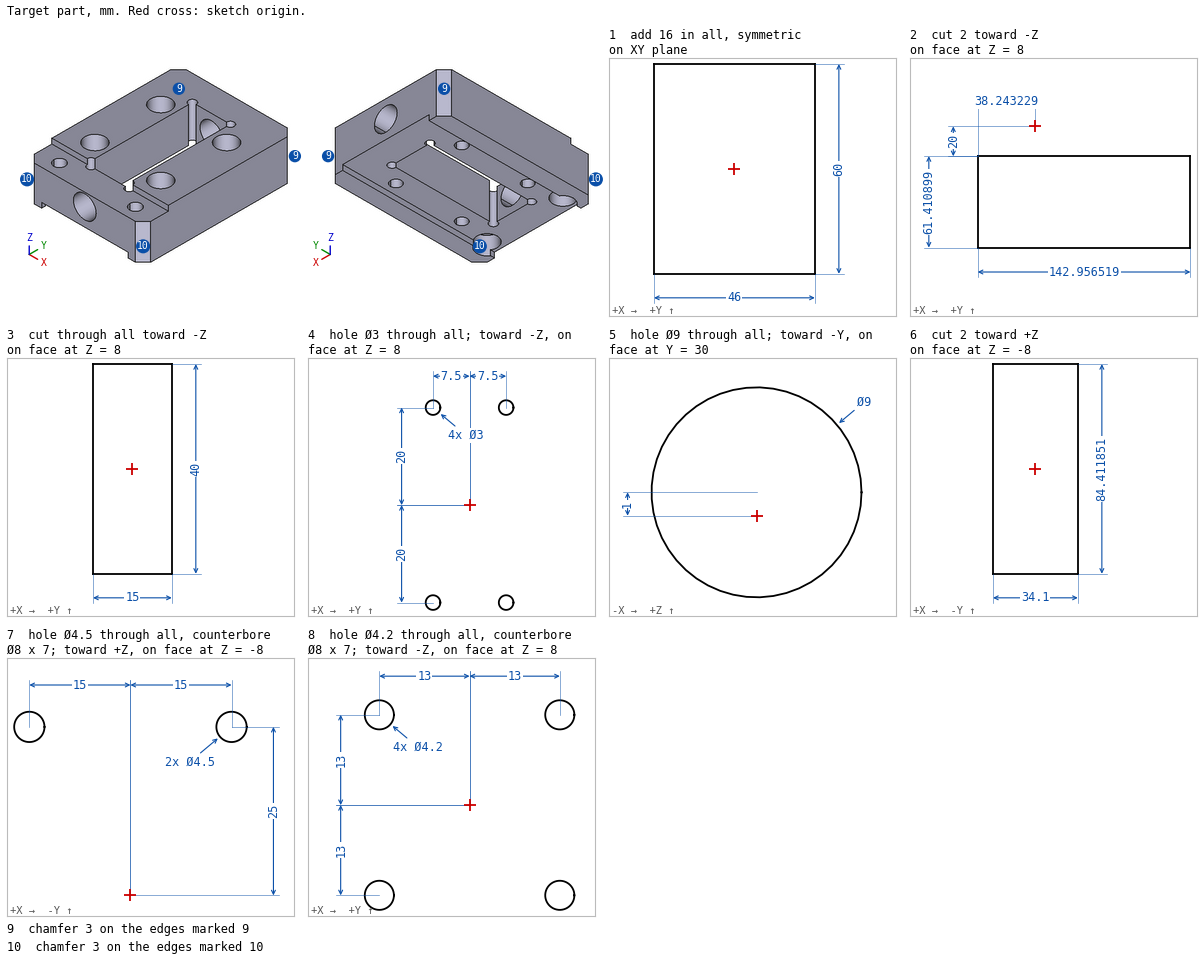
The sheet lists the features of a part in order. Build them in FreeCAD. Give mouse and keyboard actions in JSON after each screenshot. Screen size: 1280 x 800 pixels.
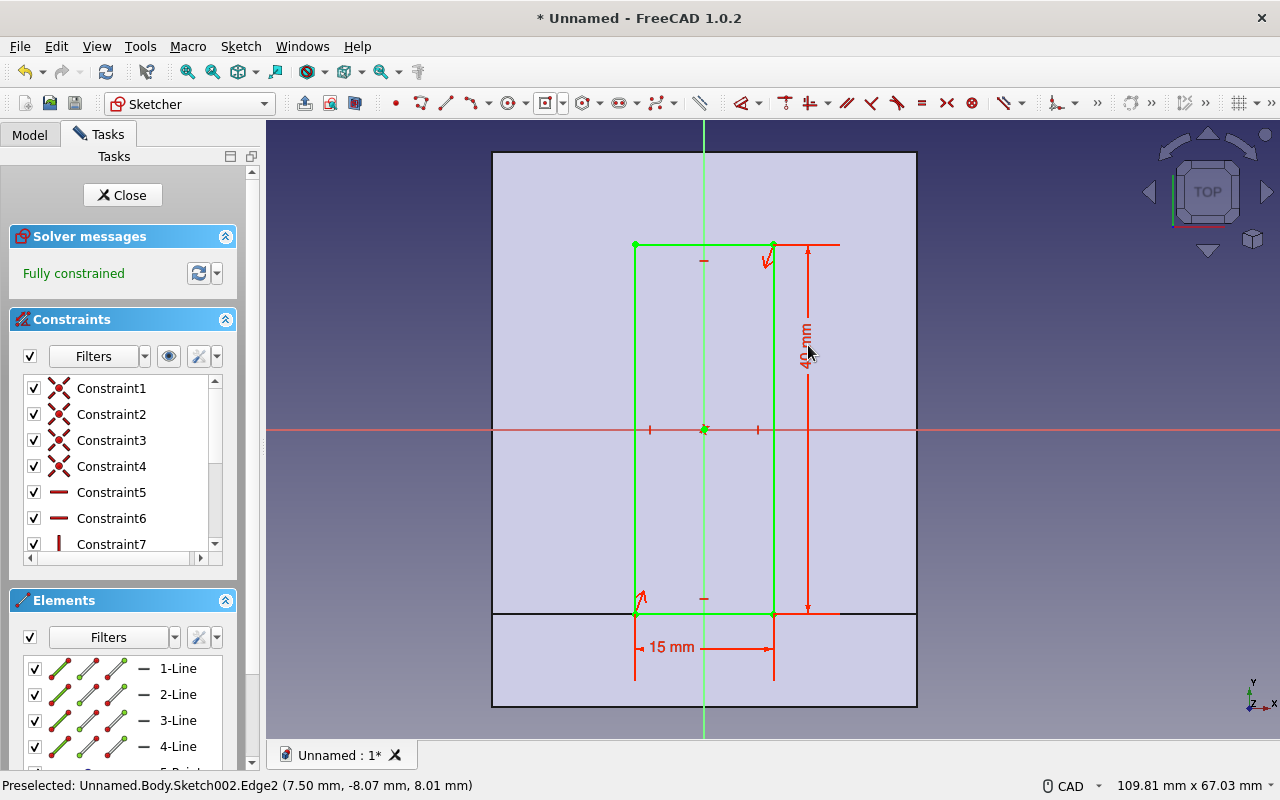
{"action": "left_click", "coordinate": [123, 195]}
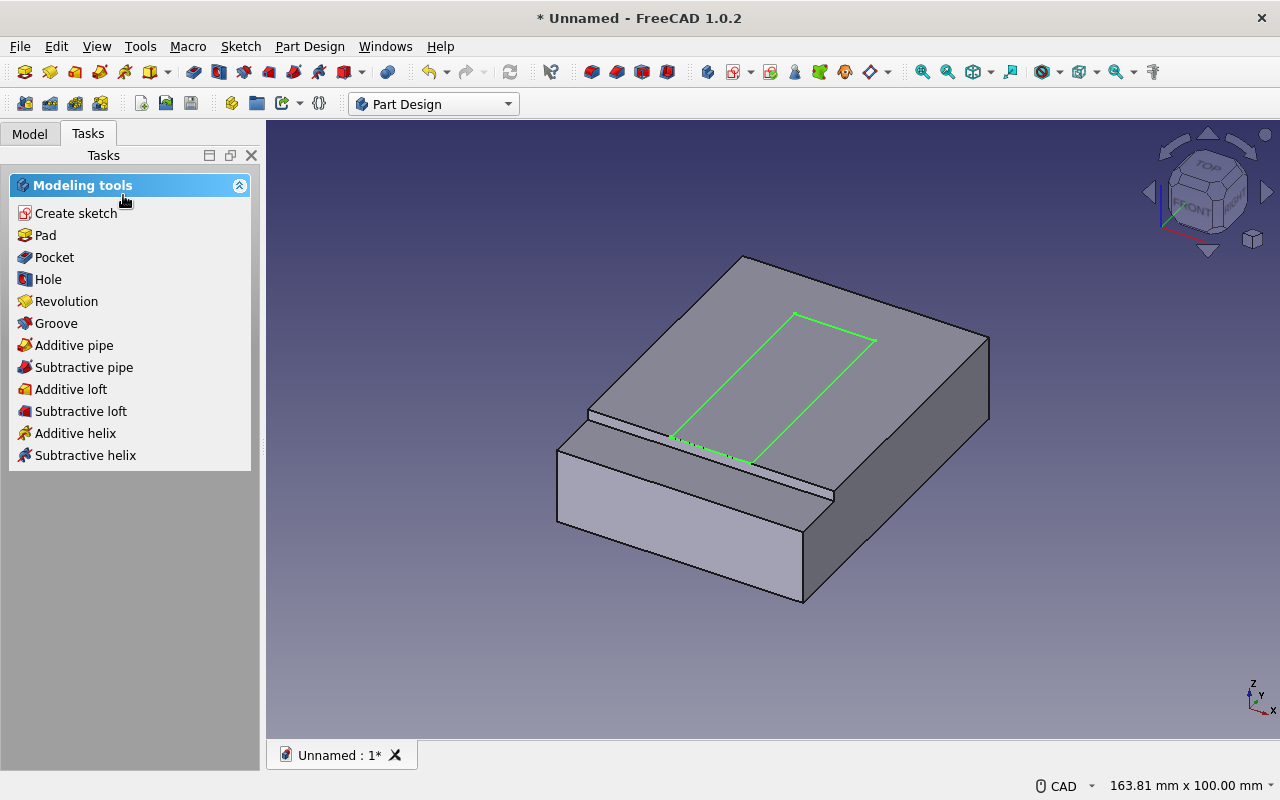
{"action": "left_click", "coordinate": [194, 72]}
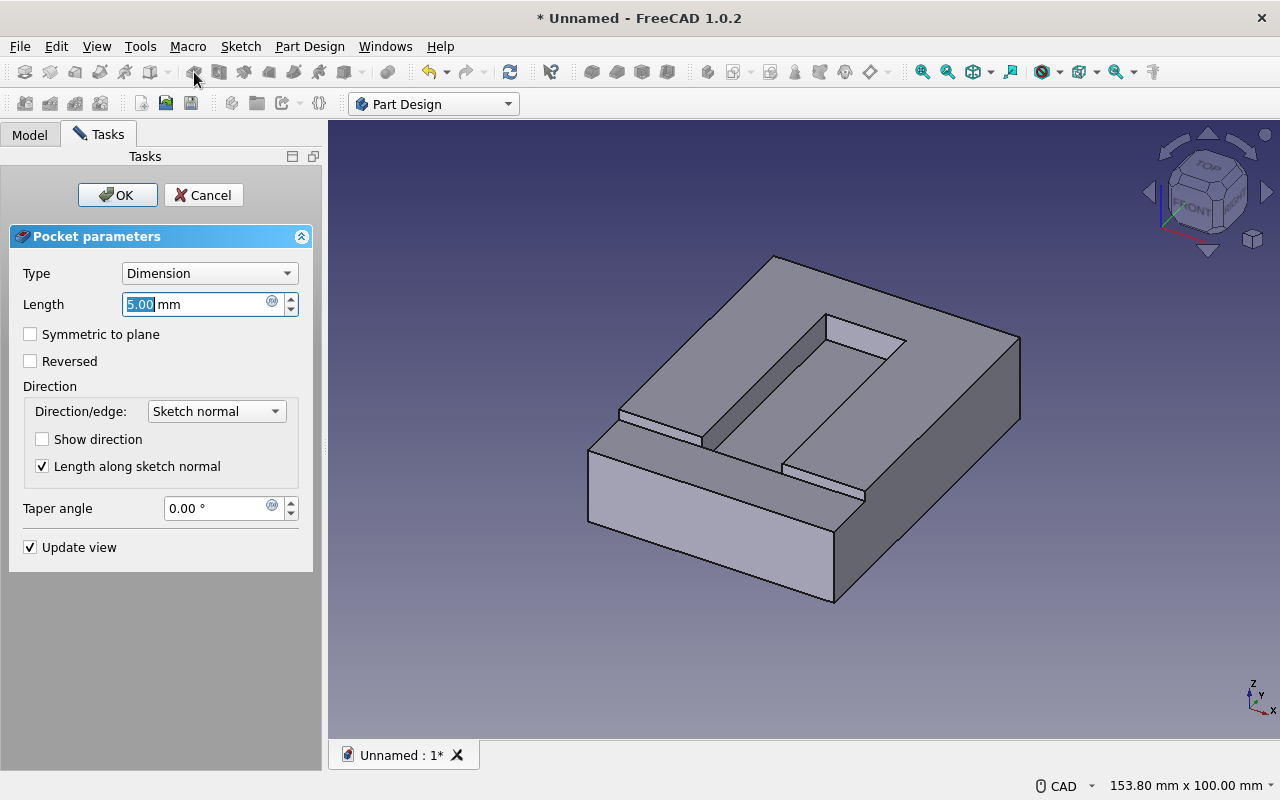
{"action": "left_click", "coordinate": [210, 274]}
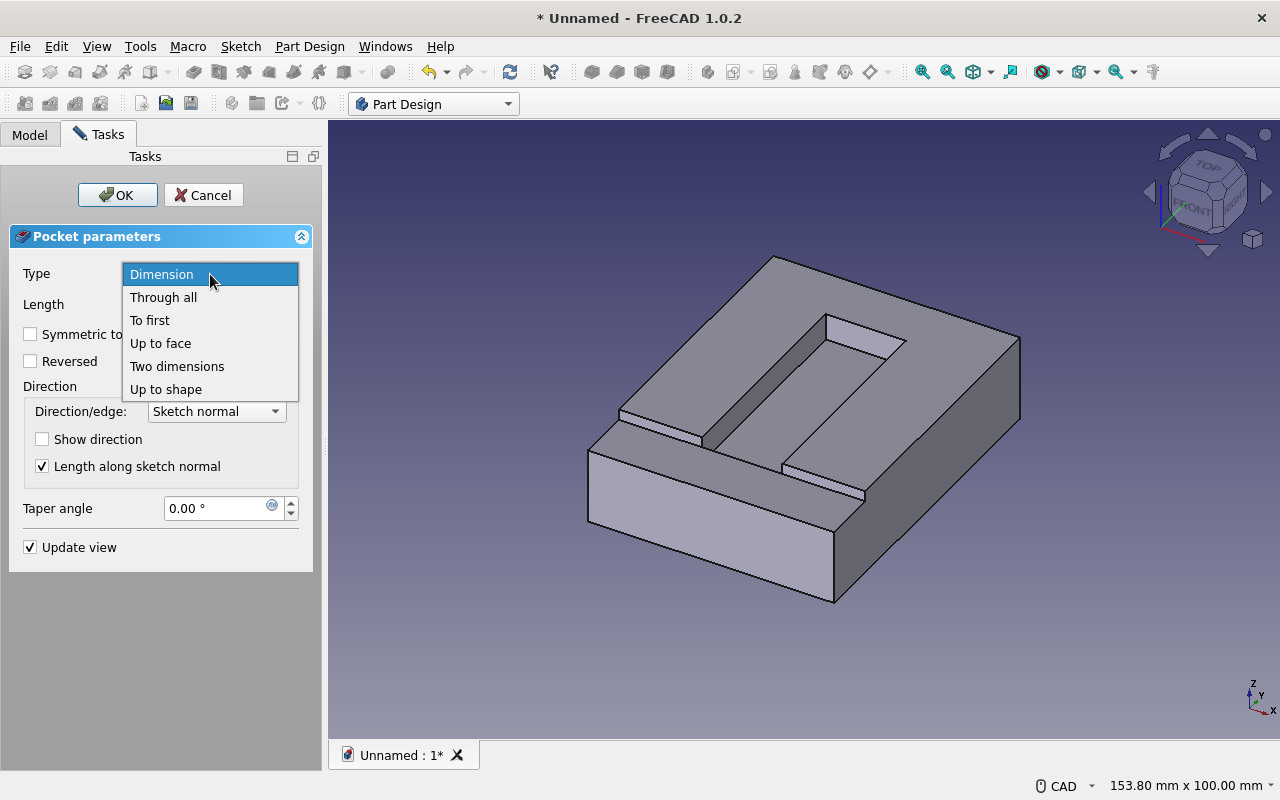
{"action": "left_click", "coordinate": [208, 298]}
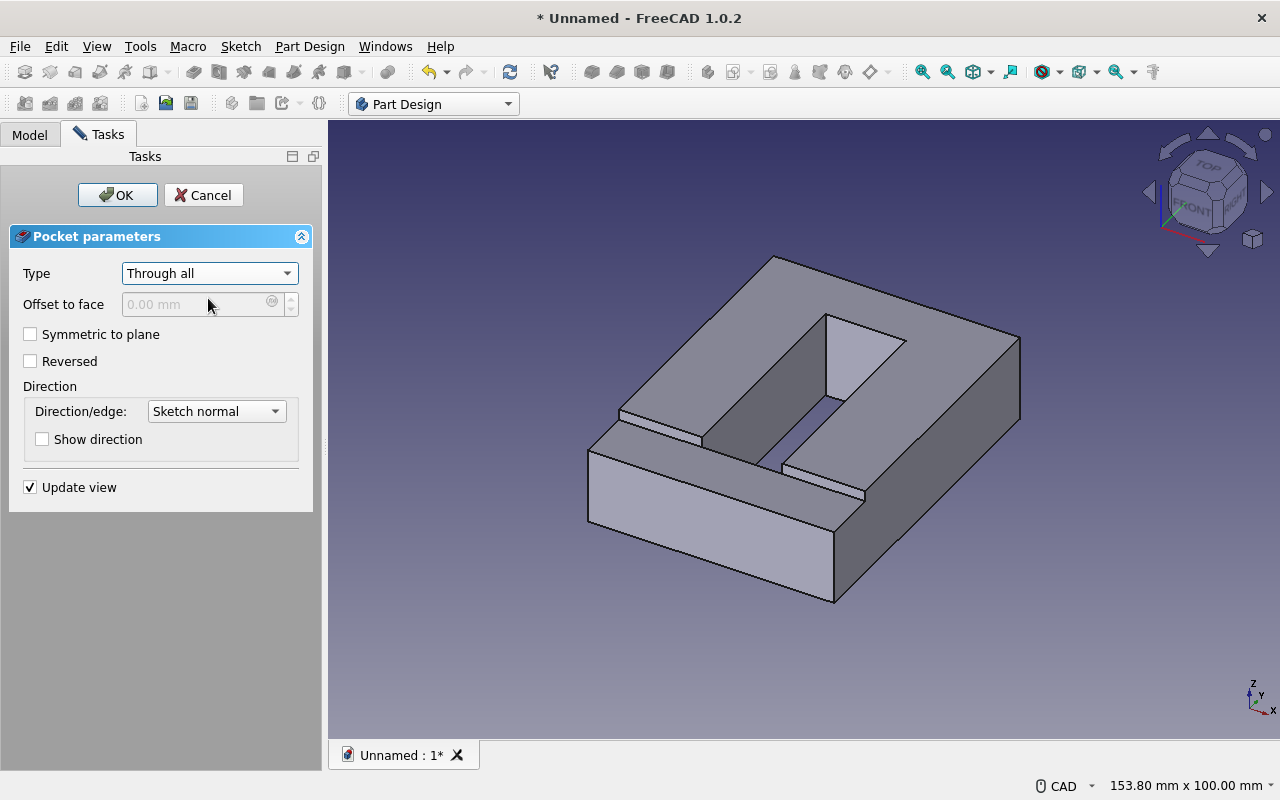
{"action": "left_click", "coordinate": [118, 195]}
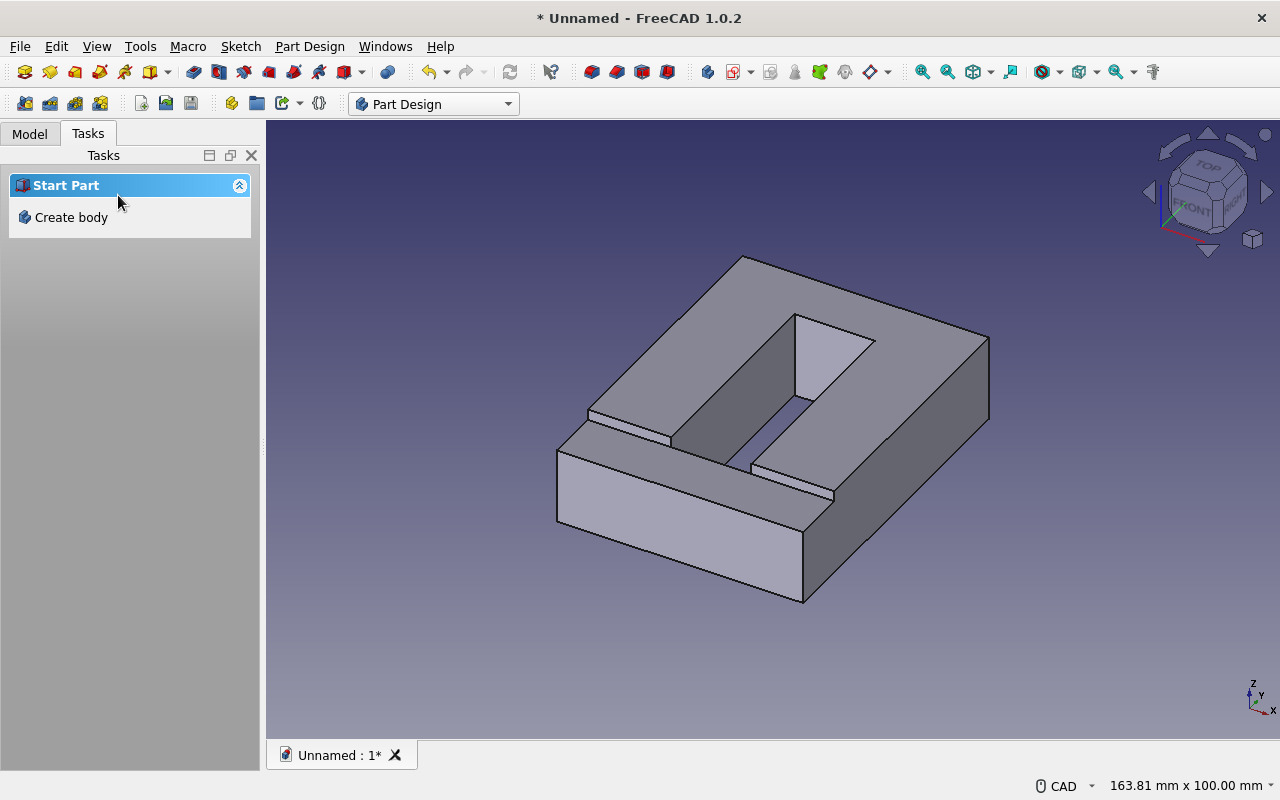
{"action": "left_click", "coordinate": [903, 352]}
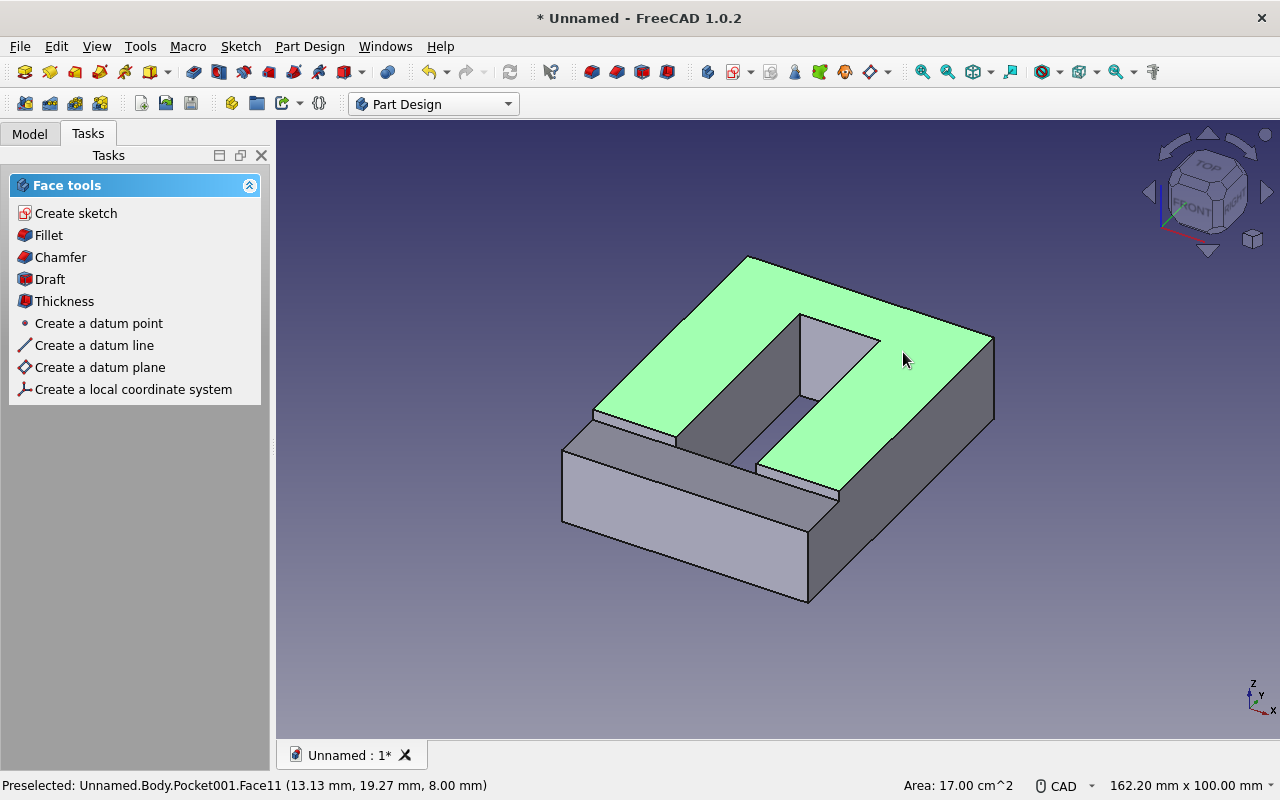
{"action": "left_click", "coordinate": [732, 72]}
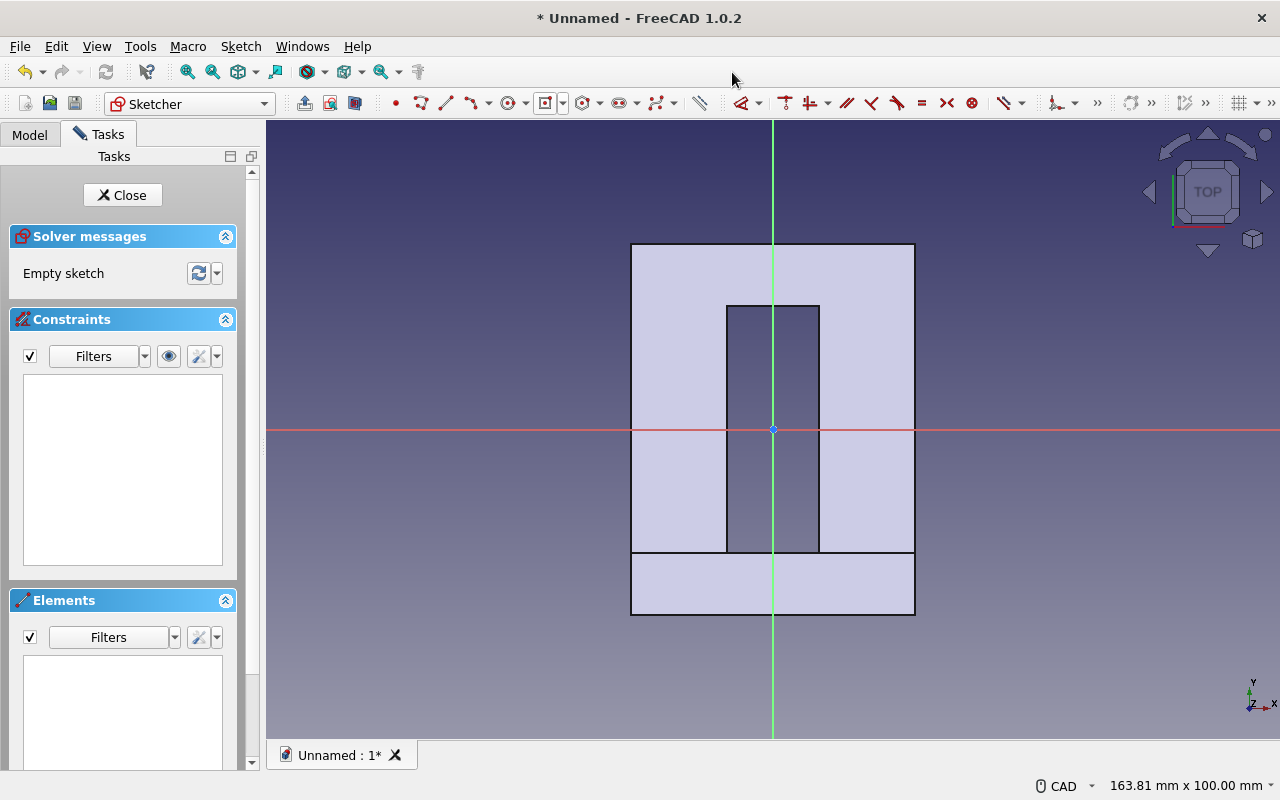
{"action": "scroll", "coordinate": [912, 429], "scroll_direction": "up", "scroll_amount": 2}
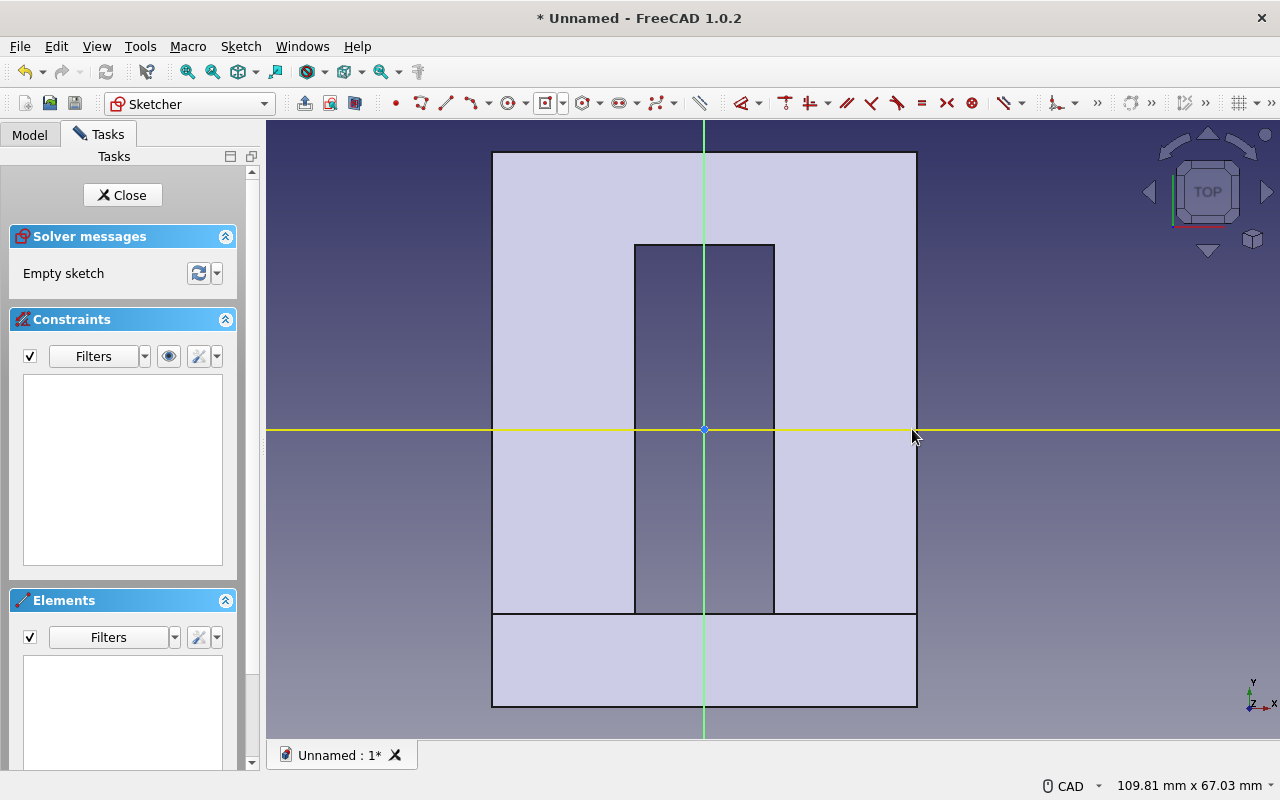
{"action": "left_click", "coordinate": [508, 104]}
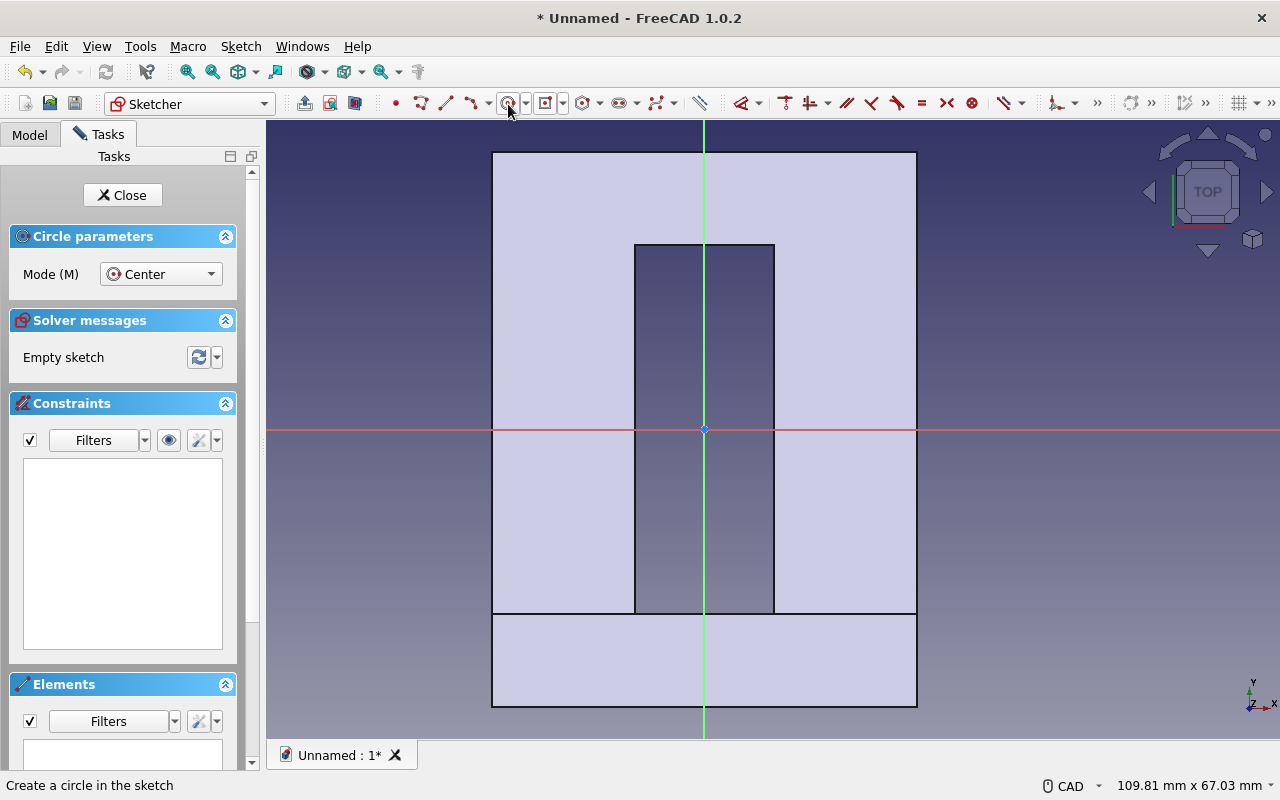
{"action": "scroll", "coordinate": [635, 245], "scroll_direction": "up", "scroll_amount": 3}